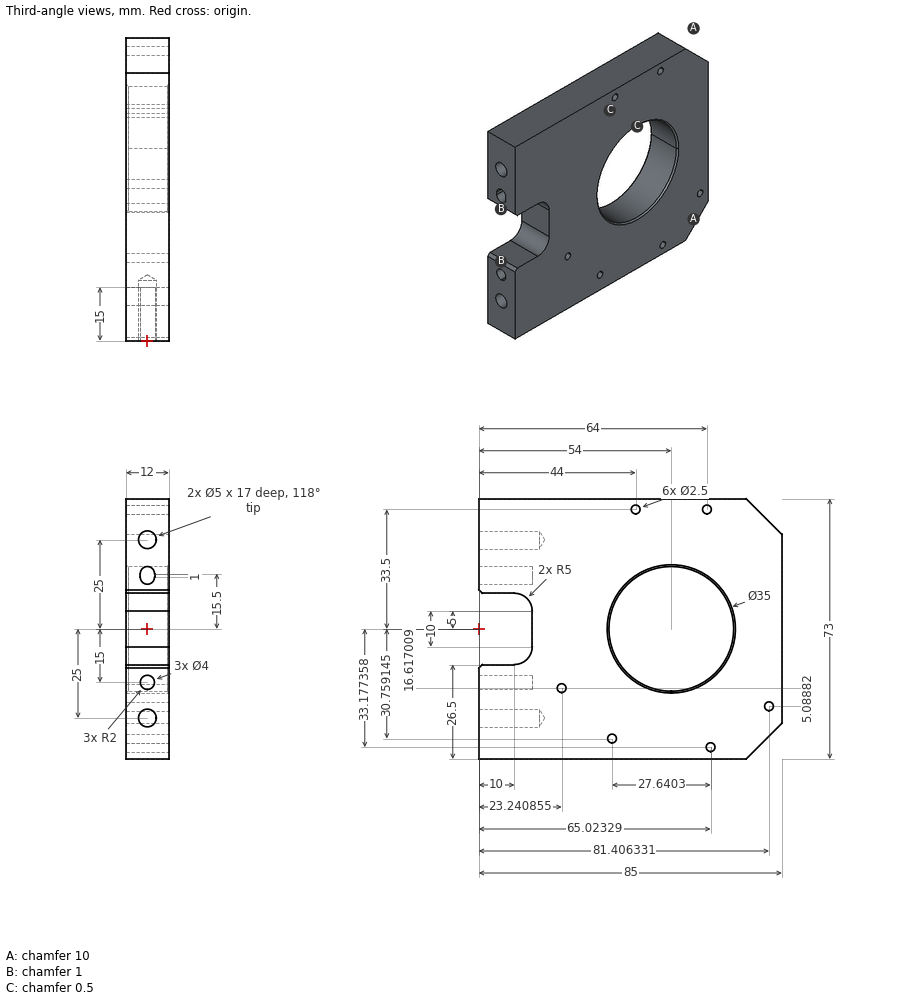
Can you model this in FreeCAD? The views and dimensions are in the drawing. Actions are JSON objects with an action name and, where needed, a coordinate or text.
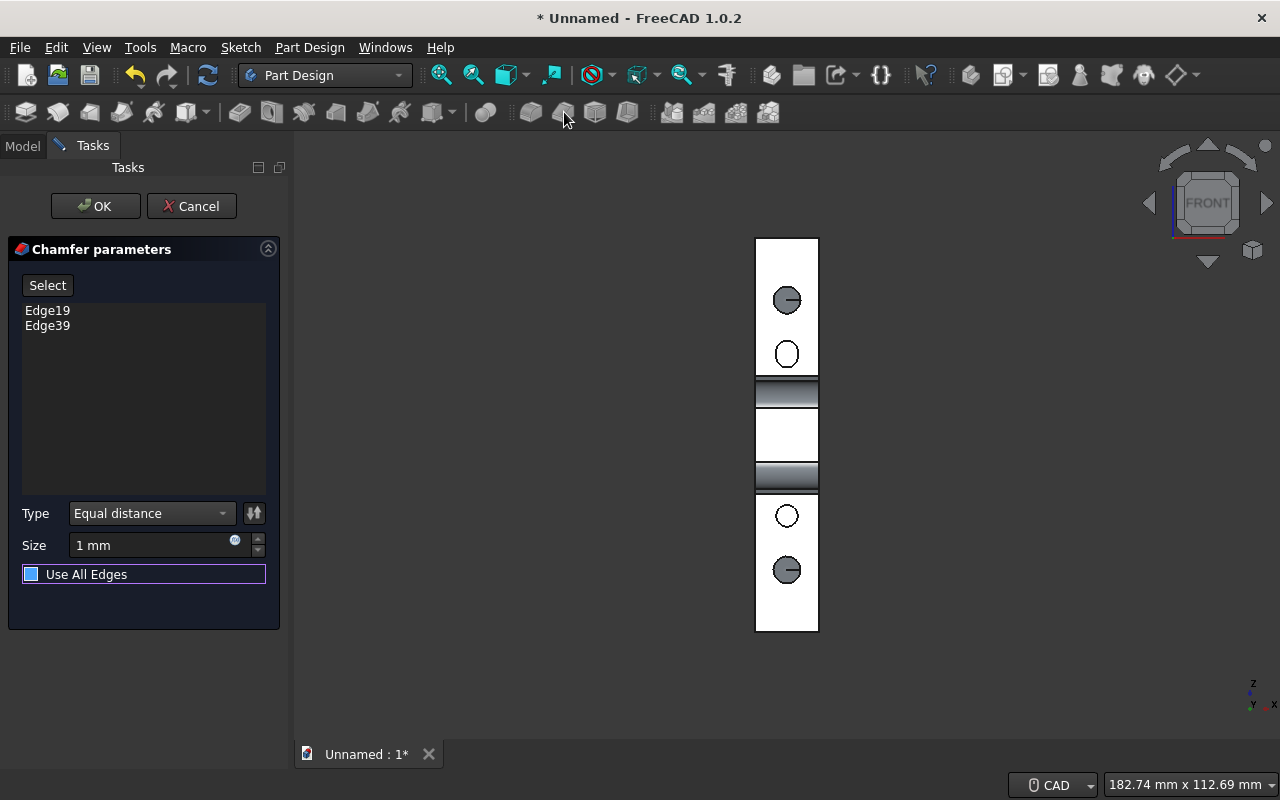
{"action": "left_click", "coordinate": [96, 206]}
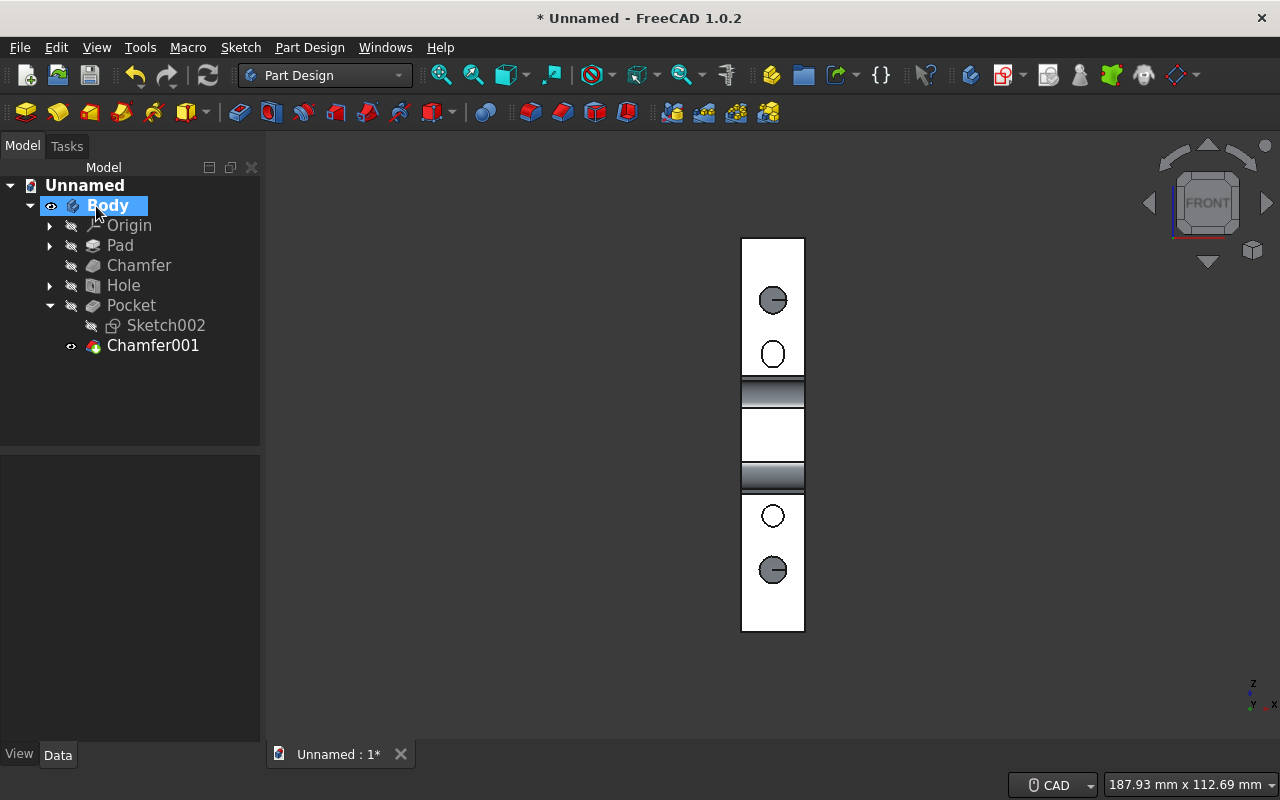
{"action": "key", "text": "6"}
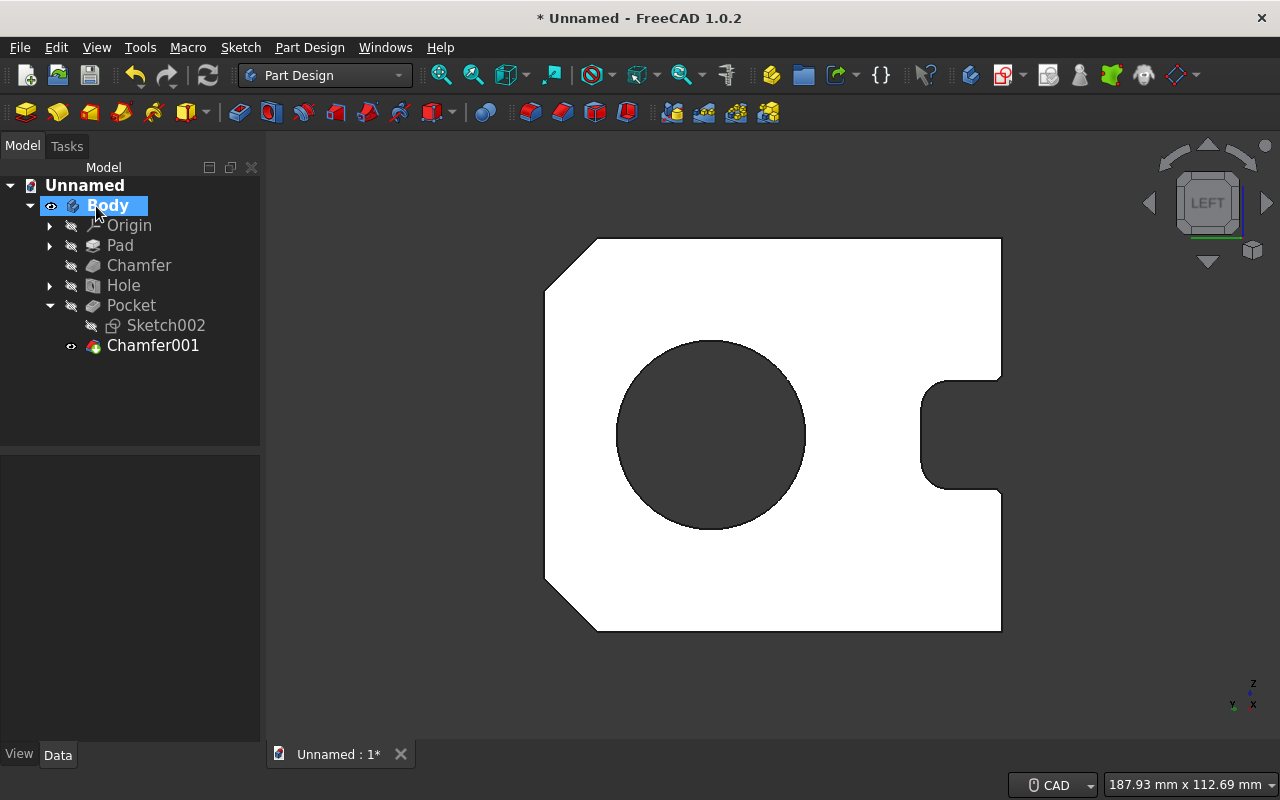
{"action": "left_click", "coordinate": [839, 547]}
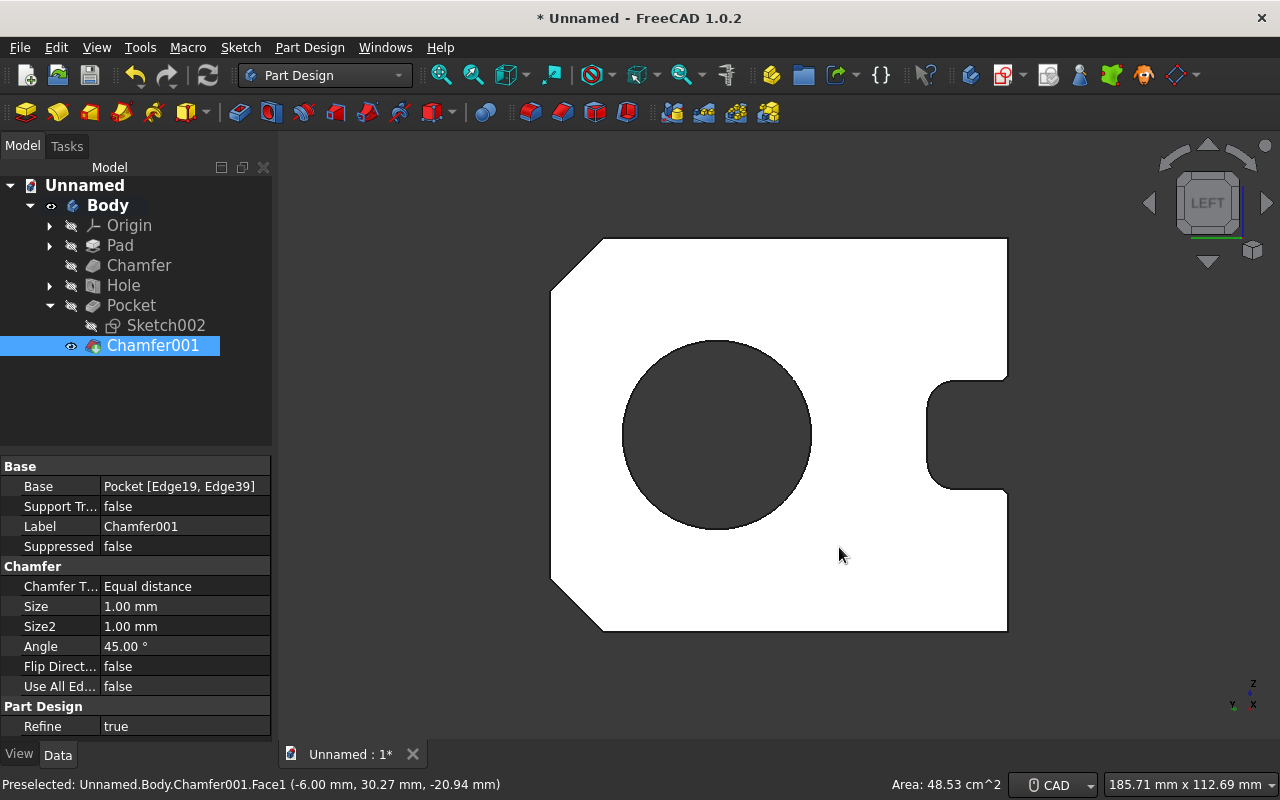
{"action": "left_click", "coordinate": [1004, 76]}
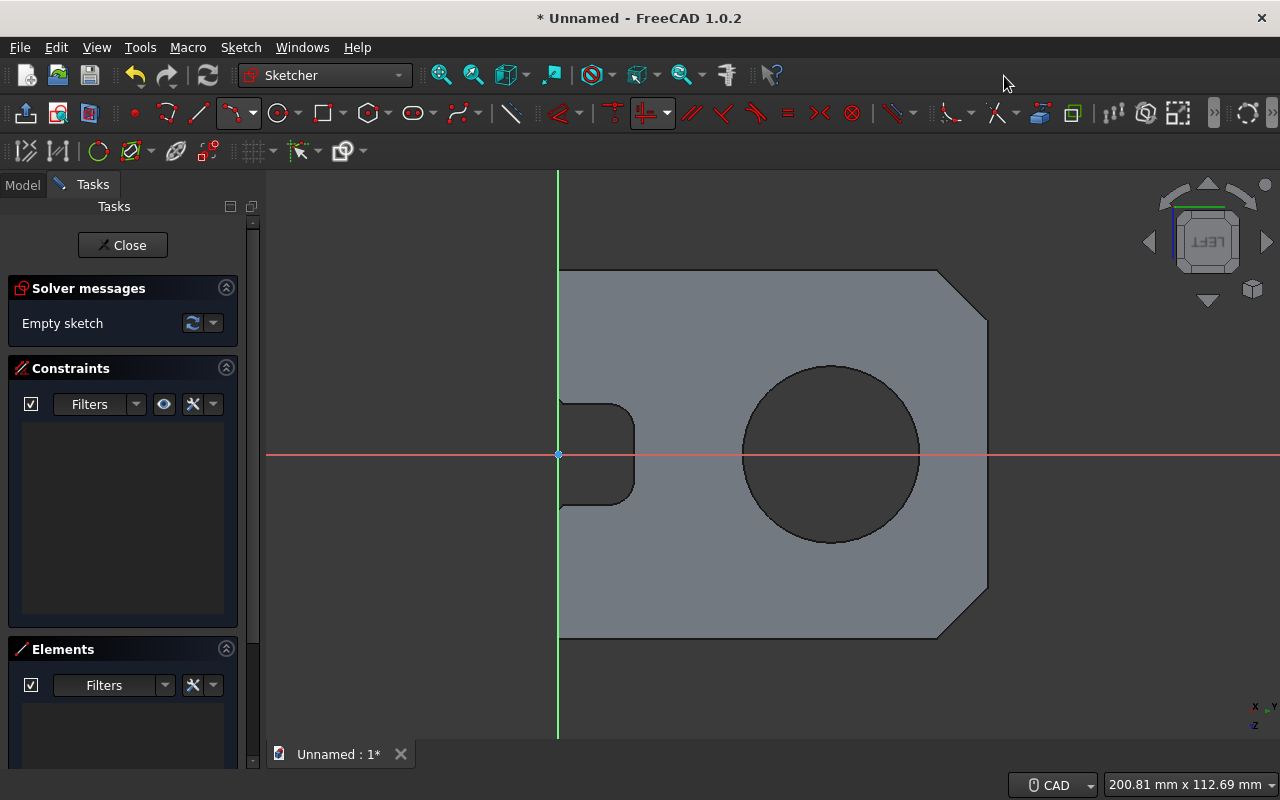
{"action": "left_click", "coordinate": [278, 114]}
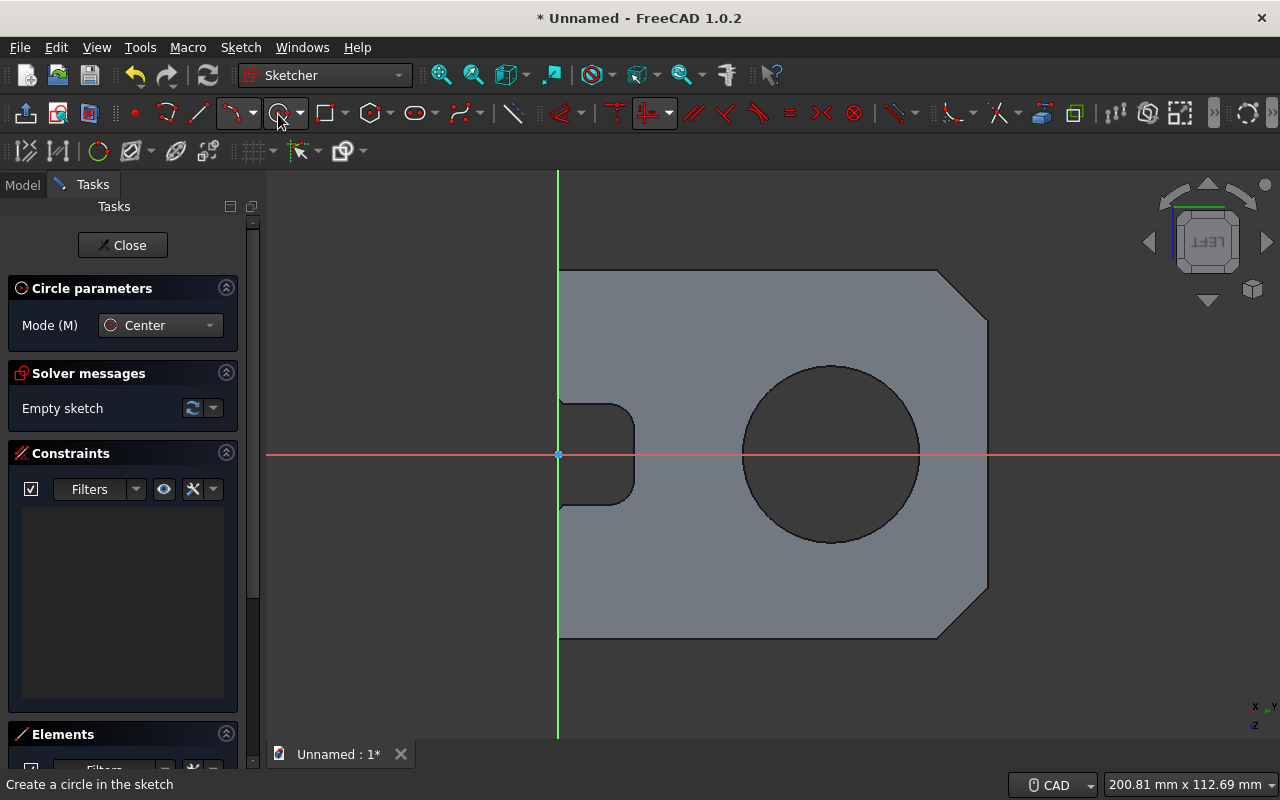
{"action": "scroll", "coordinate": [781, 624], "scroll_direction": "up", "scroll_amount": 7}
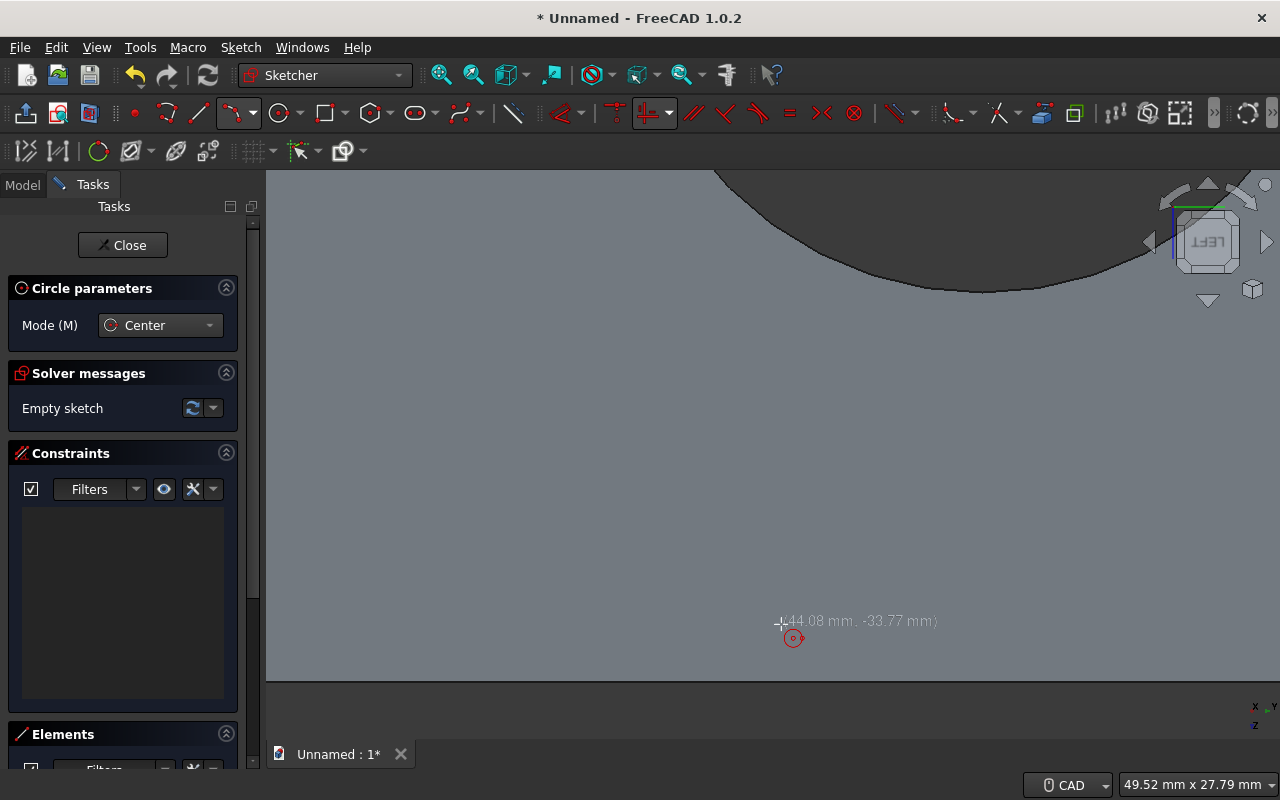
{"action": "scroll", "coordinate": [698, 624], "scroll_direction": "down", "scroll_amount": 7}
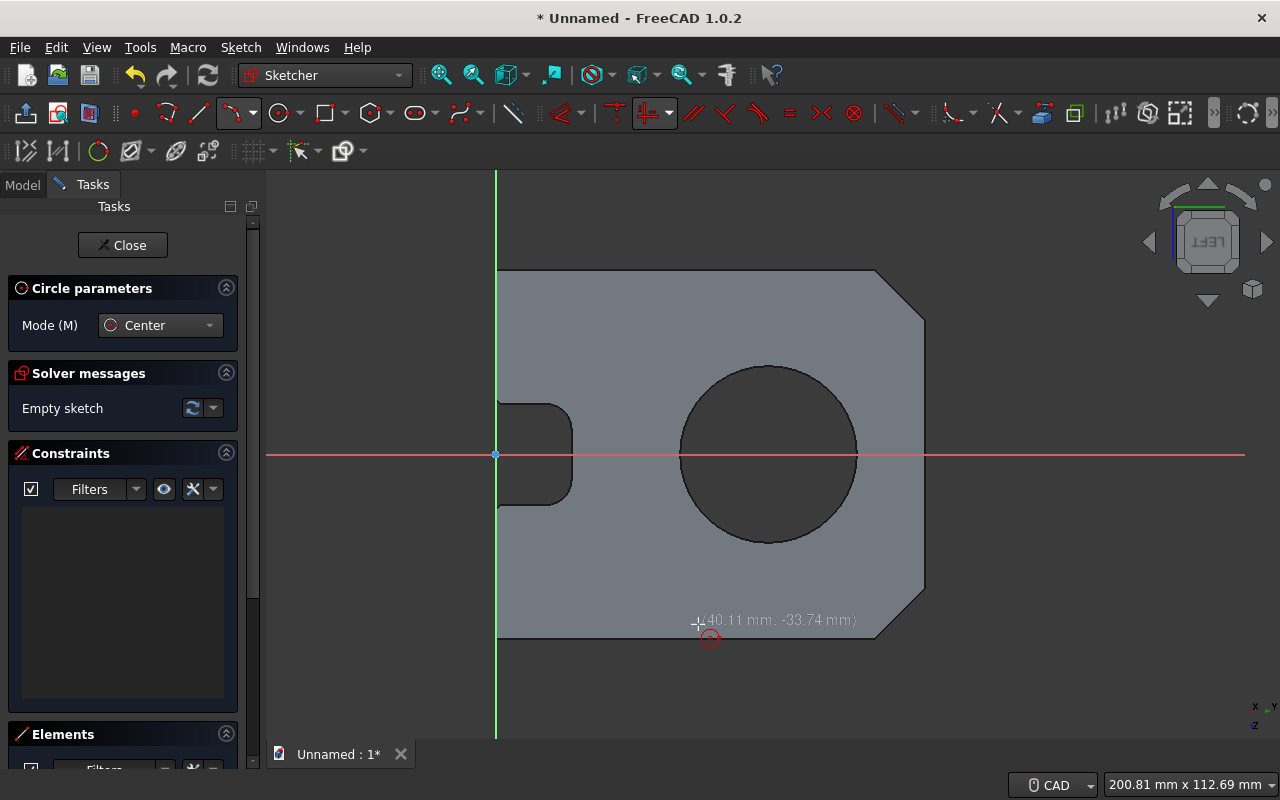
{"action": "left_click", "coordinate": [718, 624]}
{"action": "mouse_move", "coordinate": [722, 619]}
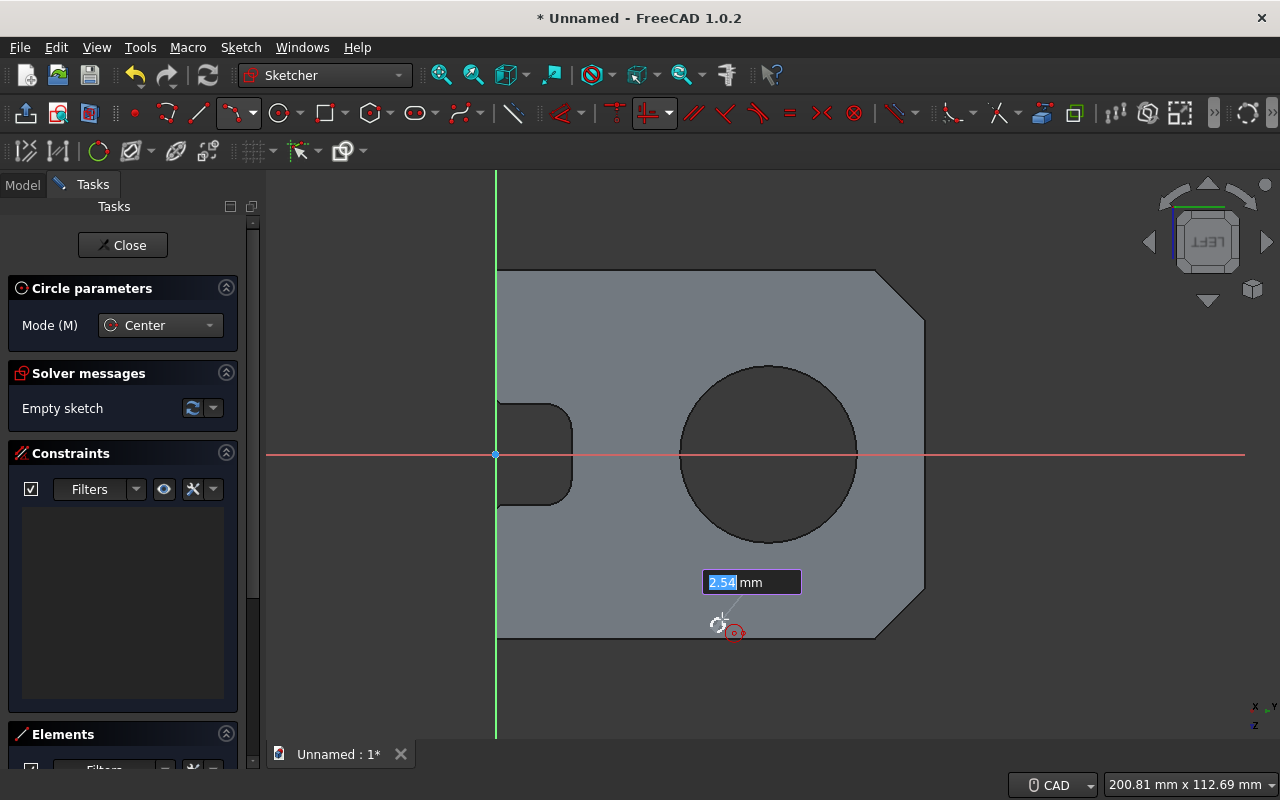
{"action": "type", "text": "2.5"}
{"action": "key", "text": "Return"}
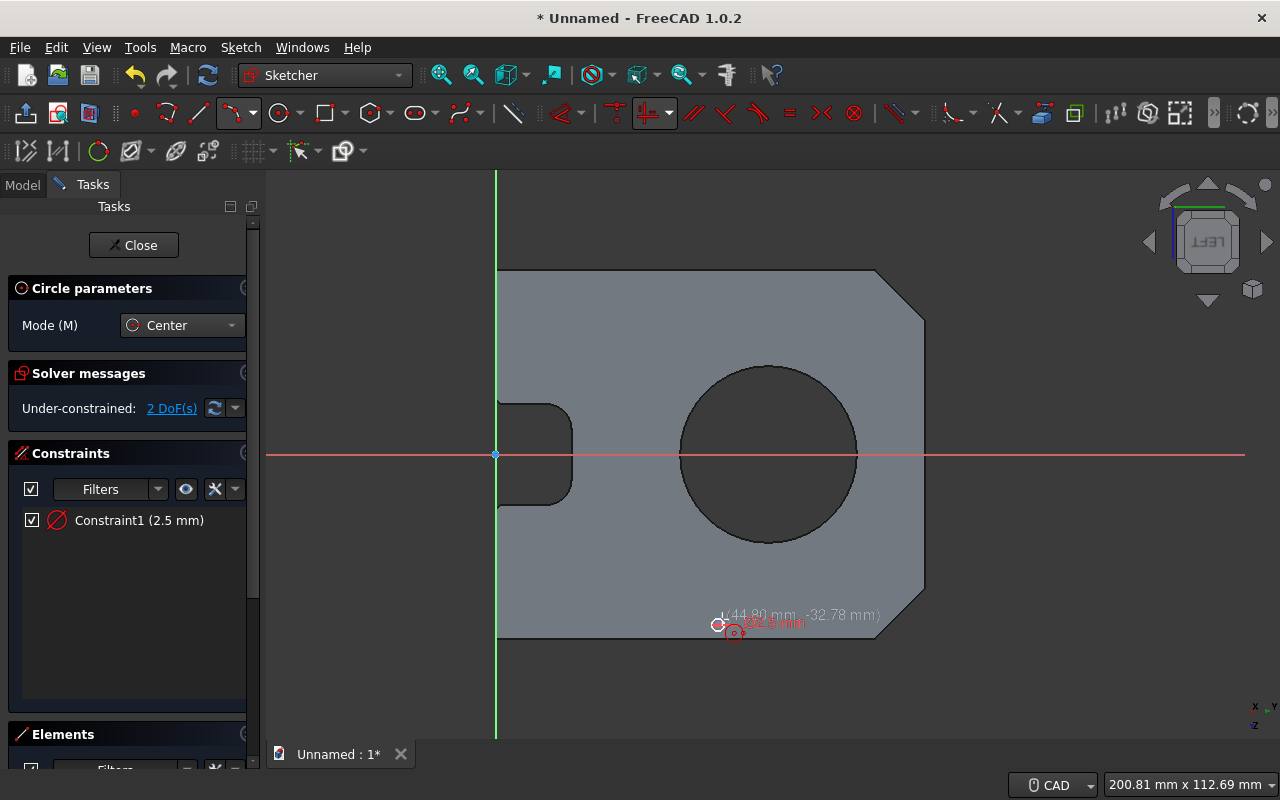
{"action": "scroll", "coordinate": [819, 624], "scroll_direction": "up", "scroll_amount": 7}